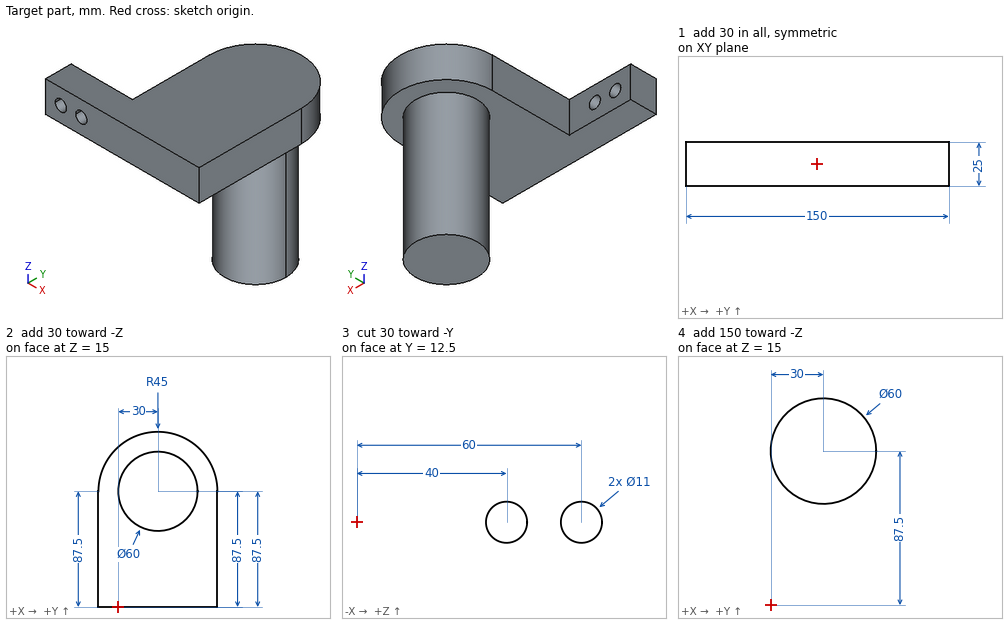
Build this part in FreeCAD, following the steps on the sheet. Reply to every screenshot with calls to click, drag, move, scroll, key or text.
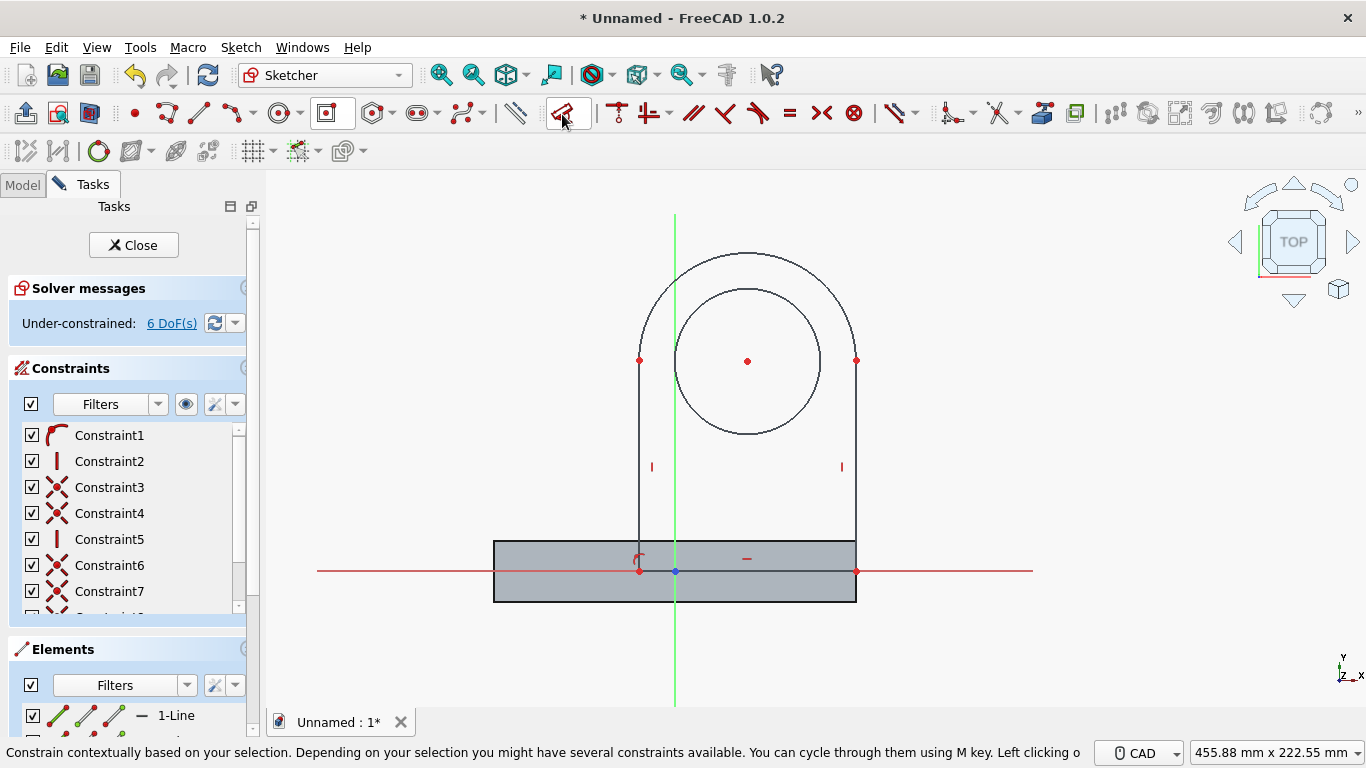
click(811, 274)
click(830, 248)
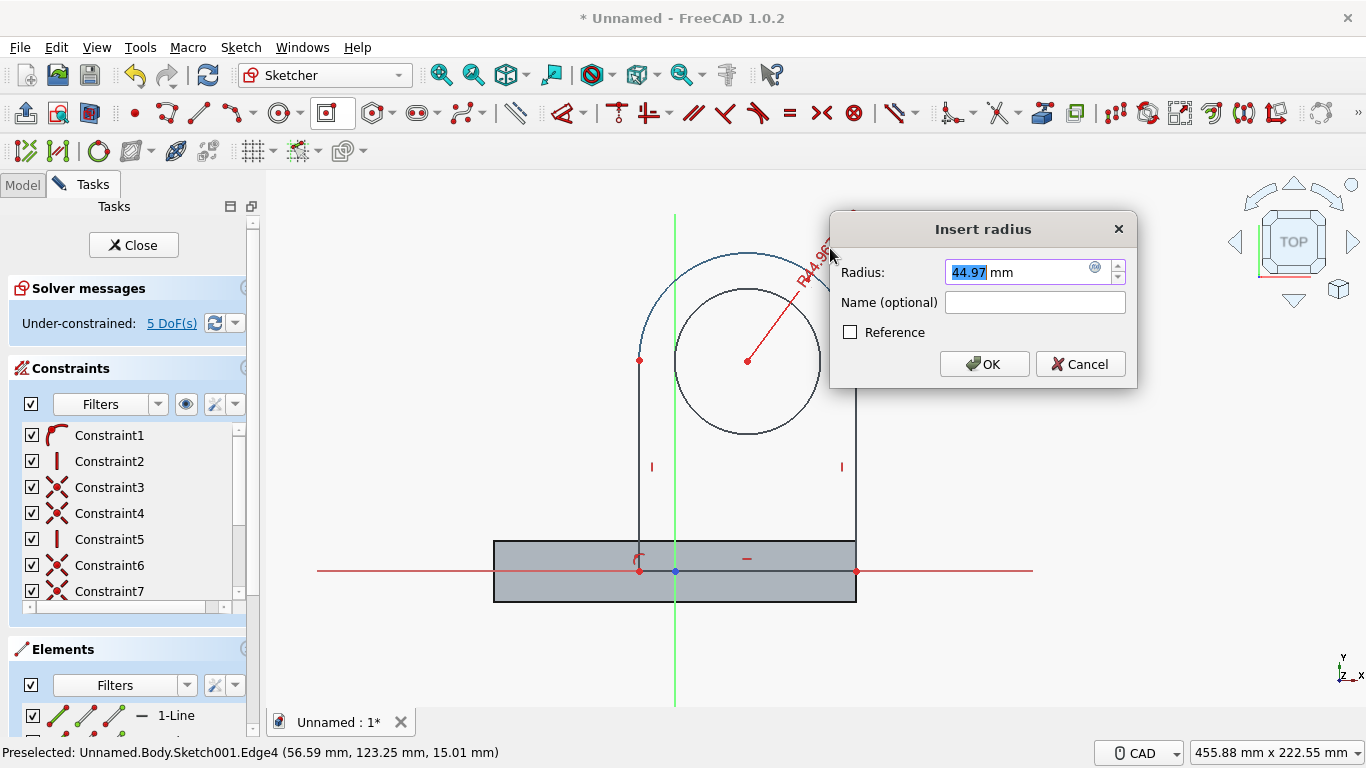
text(45)
key(Return)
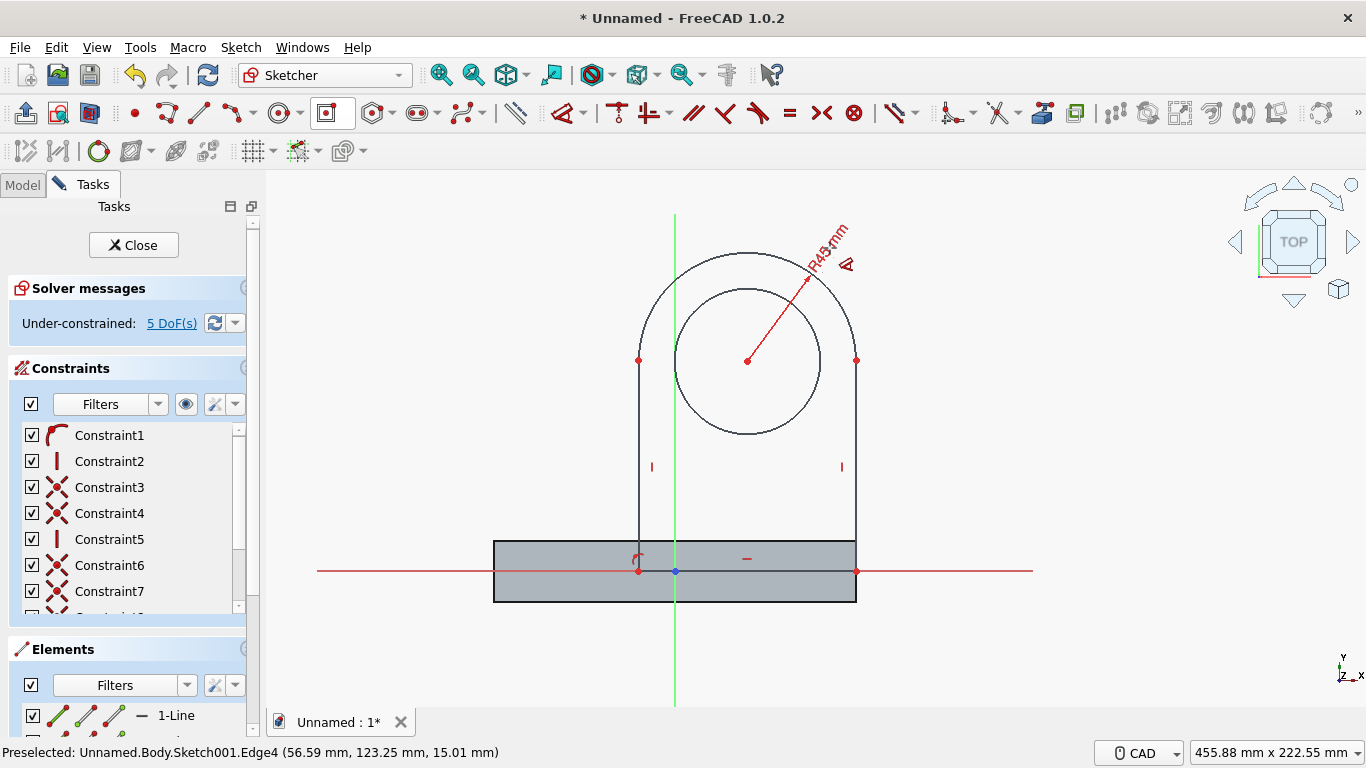
click(799, 310)
click(822, 436)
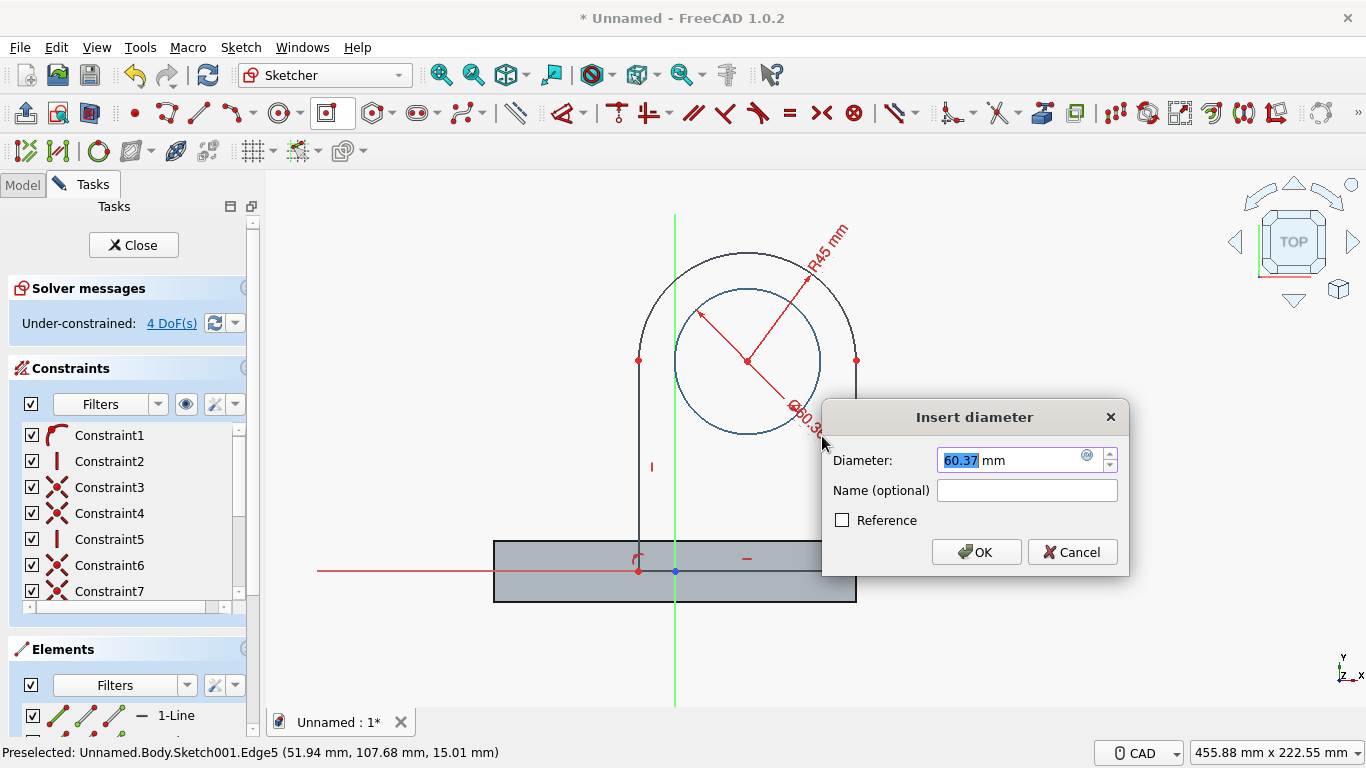
text(60)
key(Return)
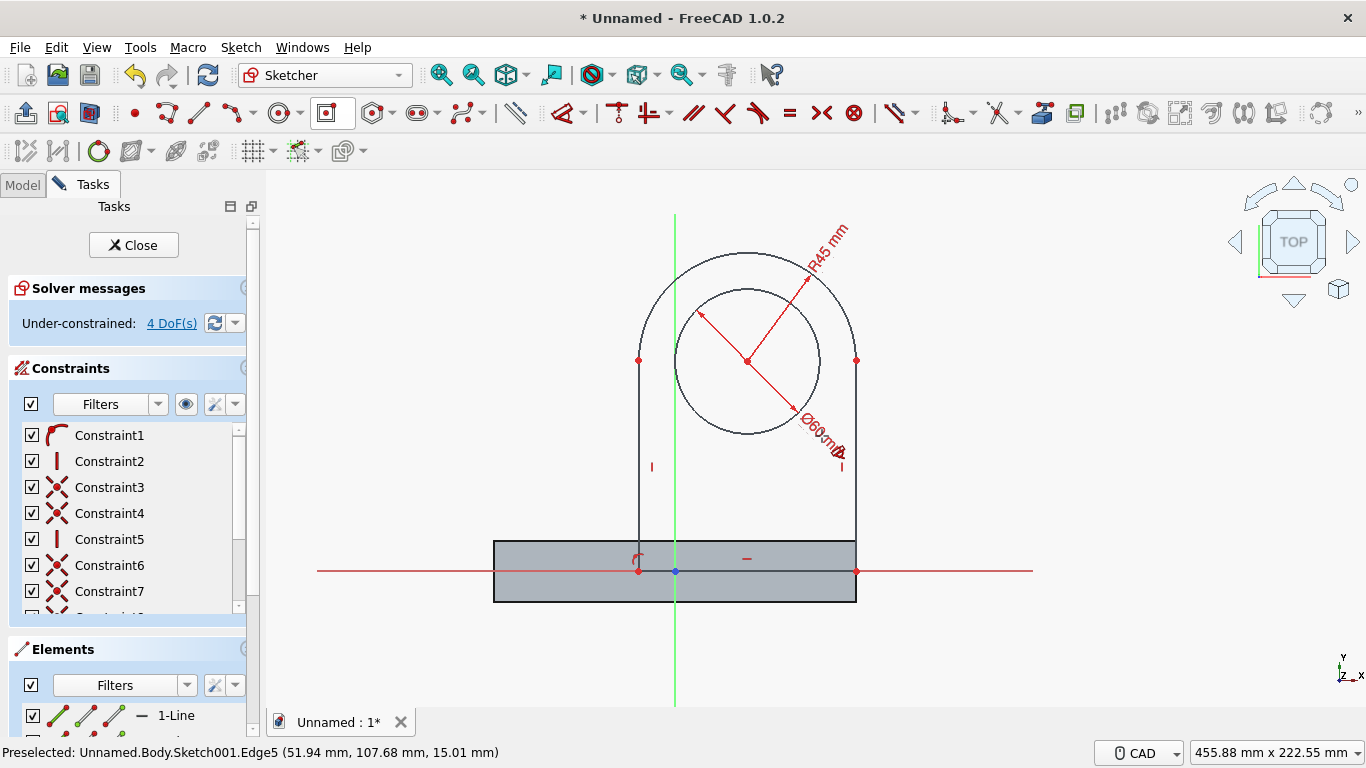
click(747, 361)
click(711, 605)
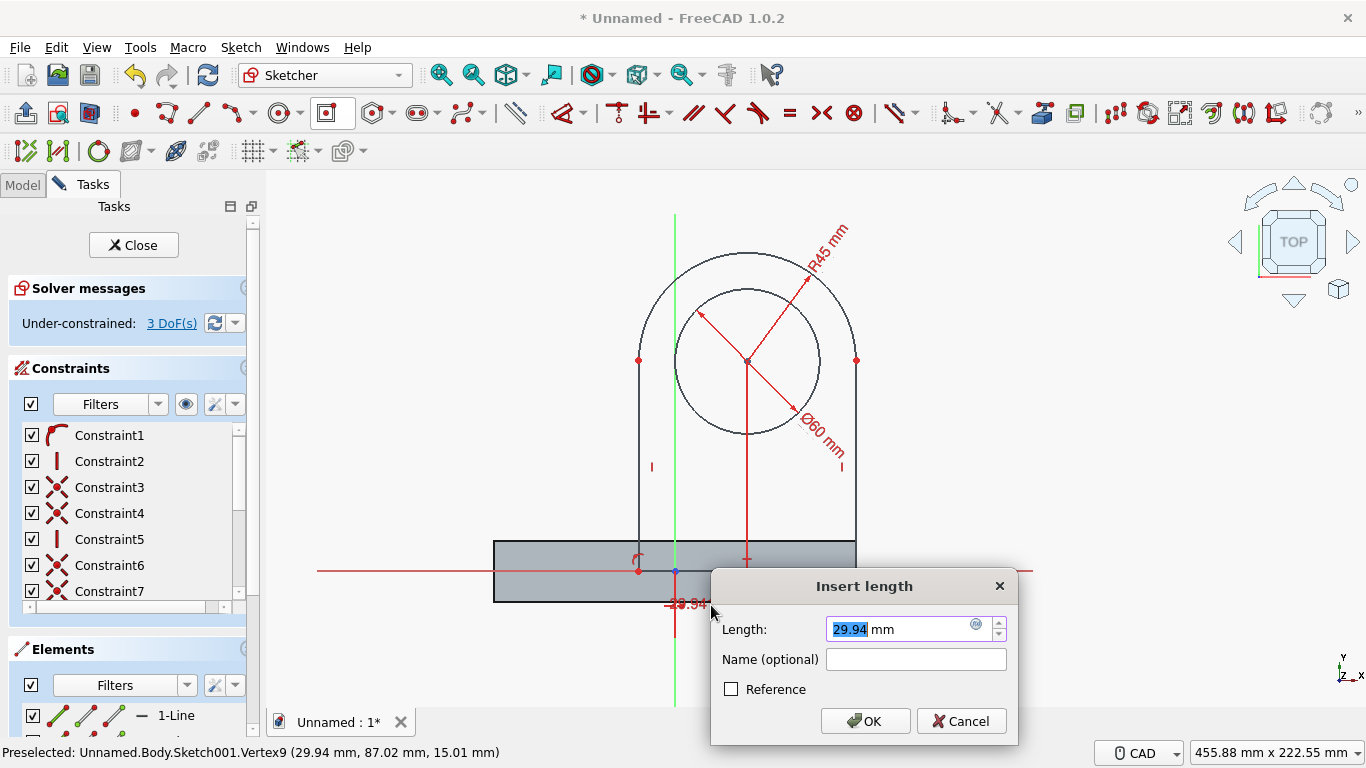
text(30)
key(Return)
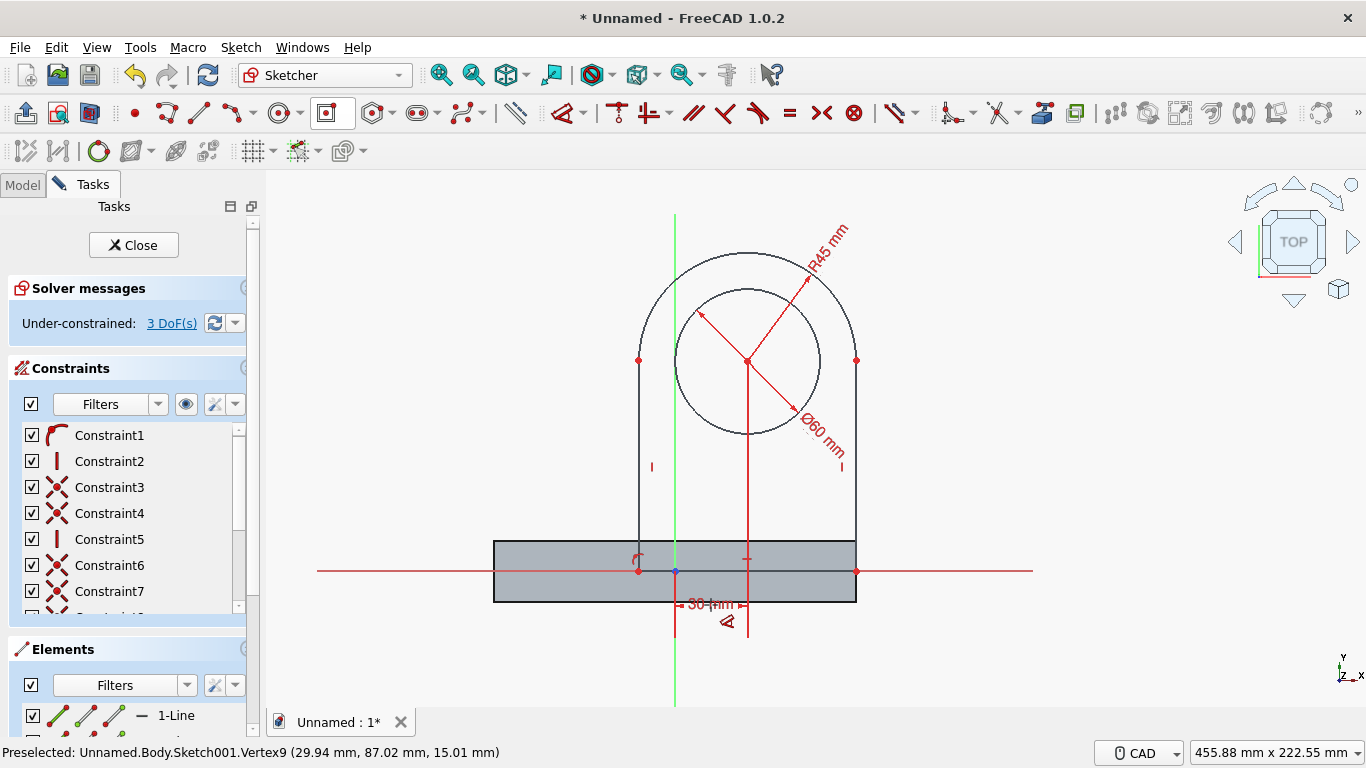
click(639, 424)
click(605, 466)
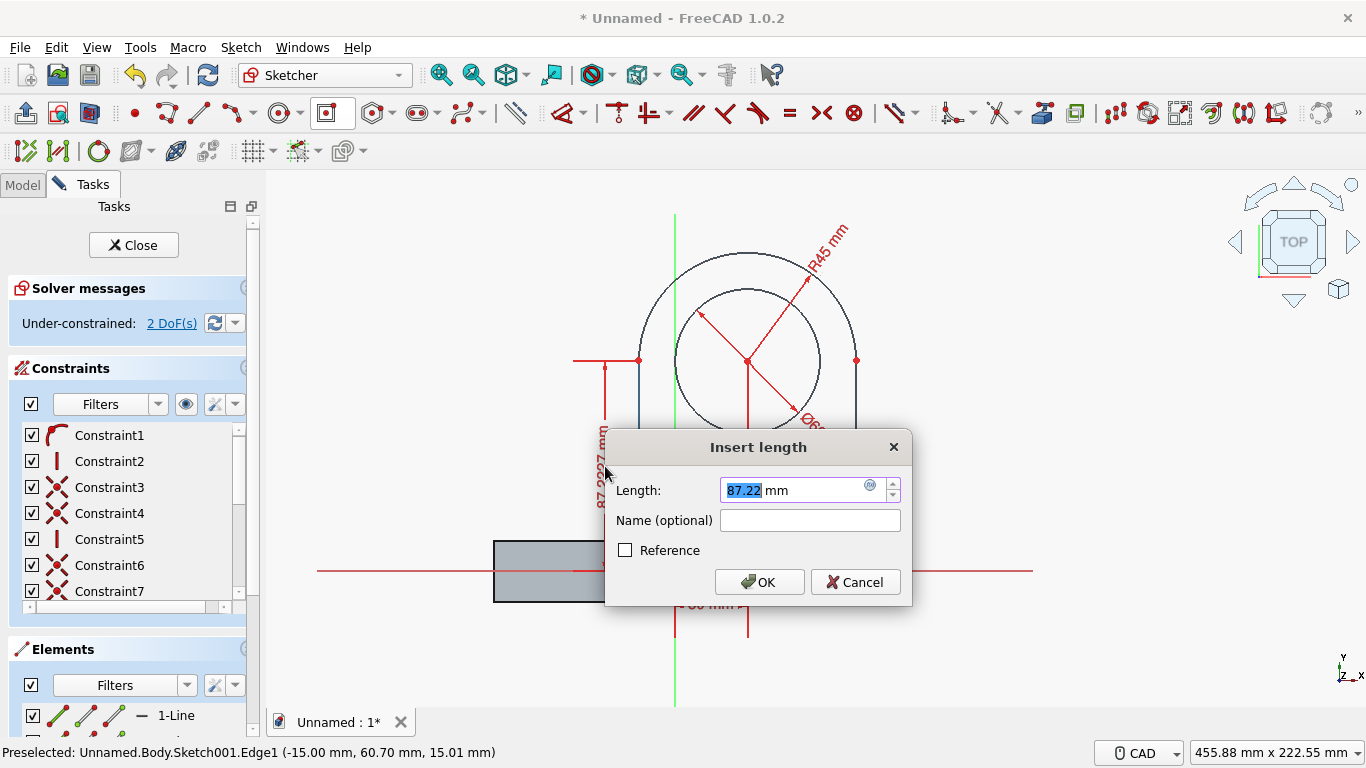
text(87.5)
key(Return)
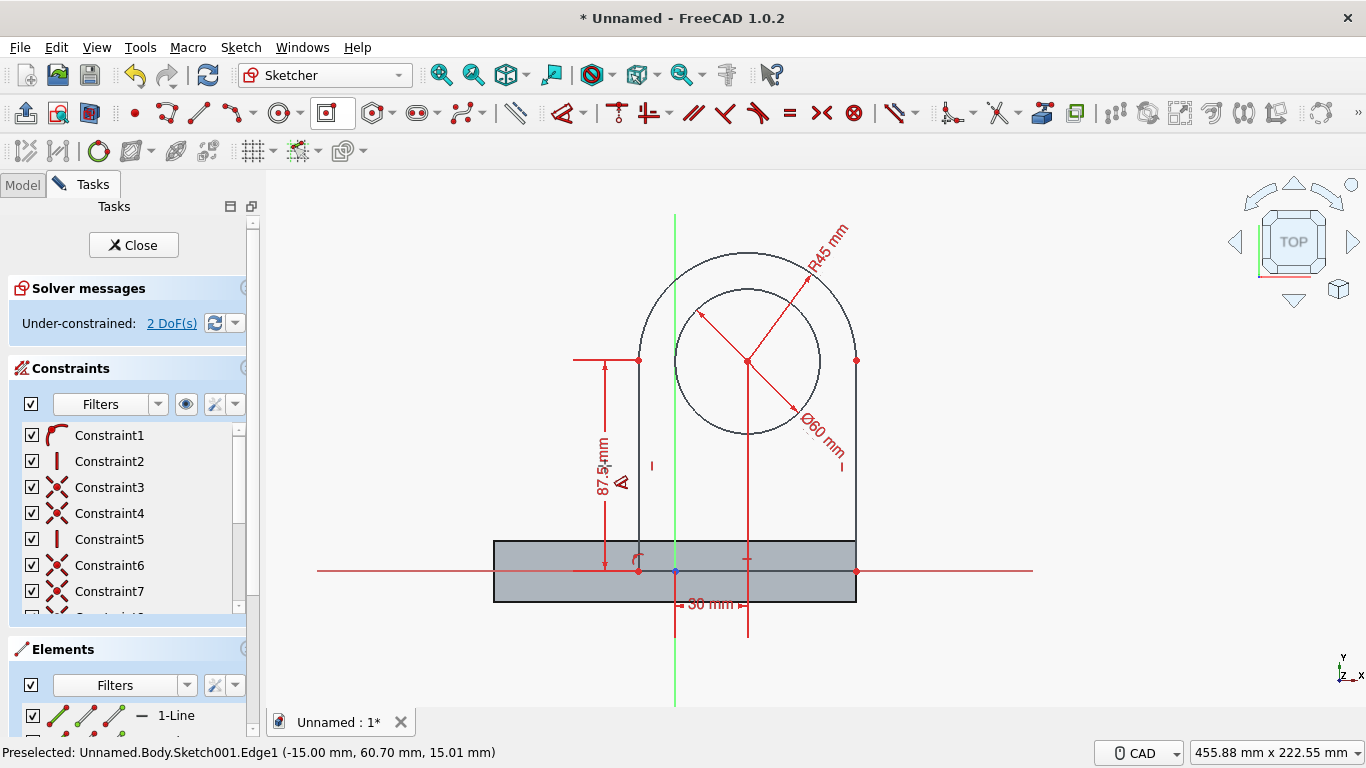
click(856, 508)
click(890, 466)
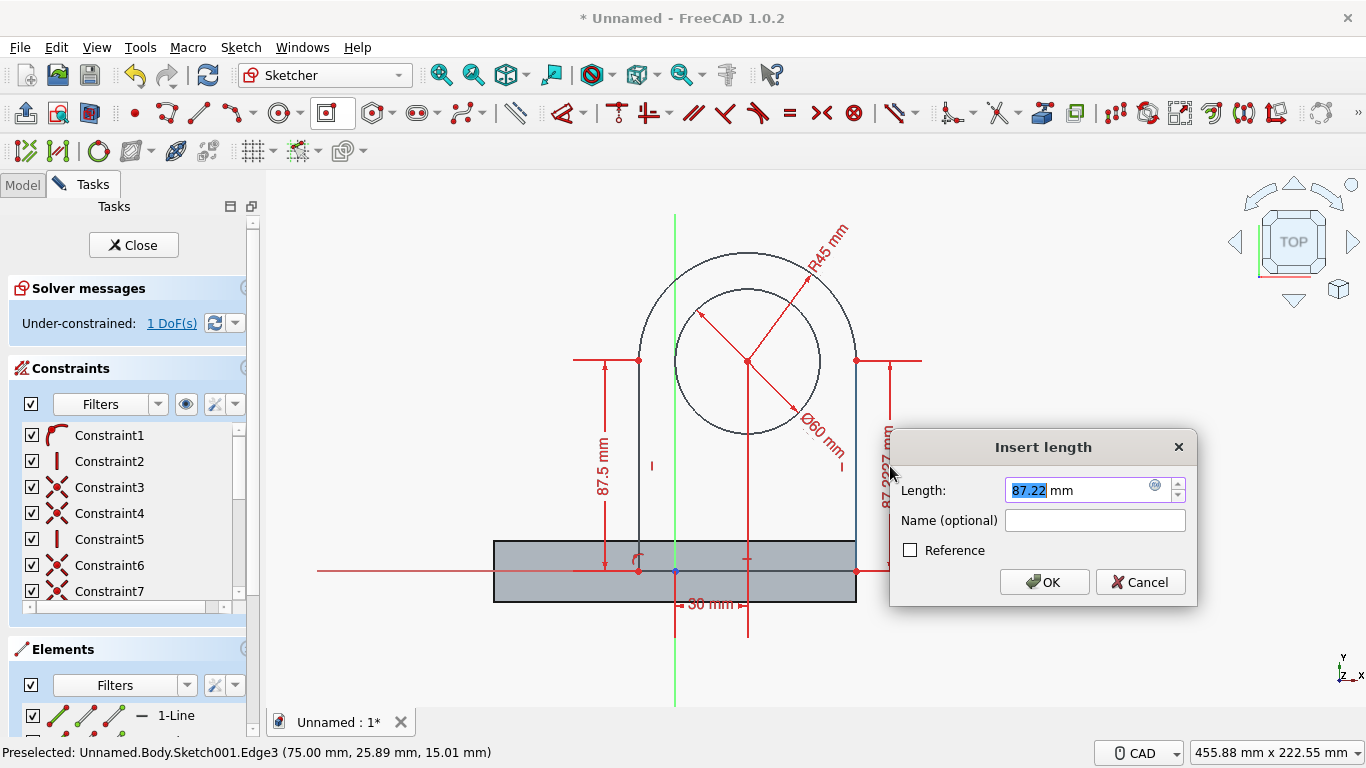
text(87.5)
key(Return)